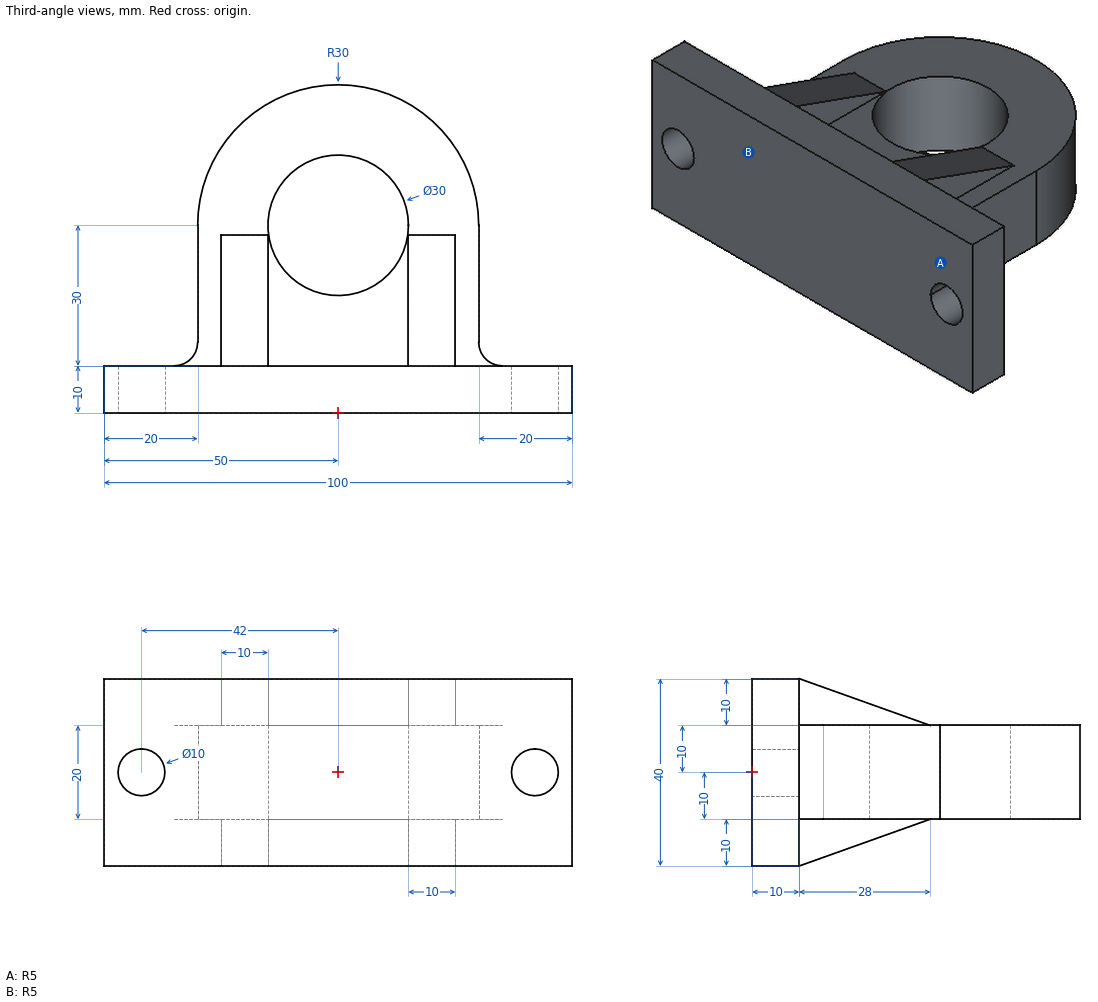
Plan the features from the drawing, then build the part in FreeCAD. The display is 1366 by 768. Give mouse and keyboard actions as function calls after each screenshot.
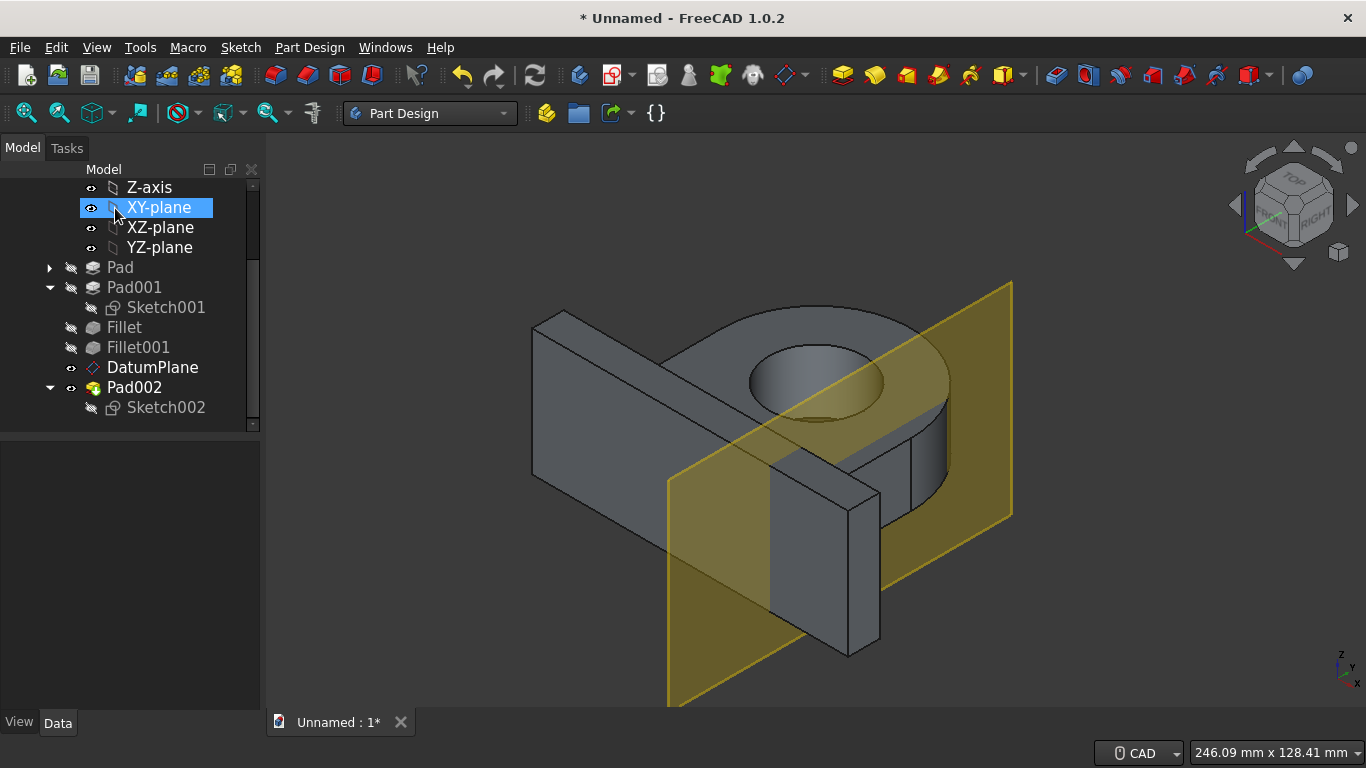
click(116, 368)
key(space)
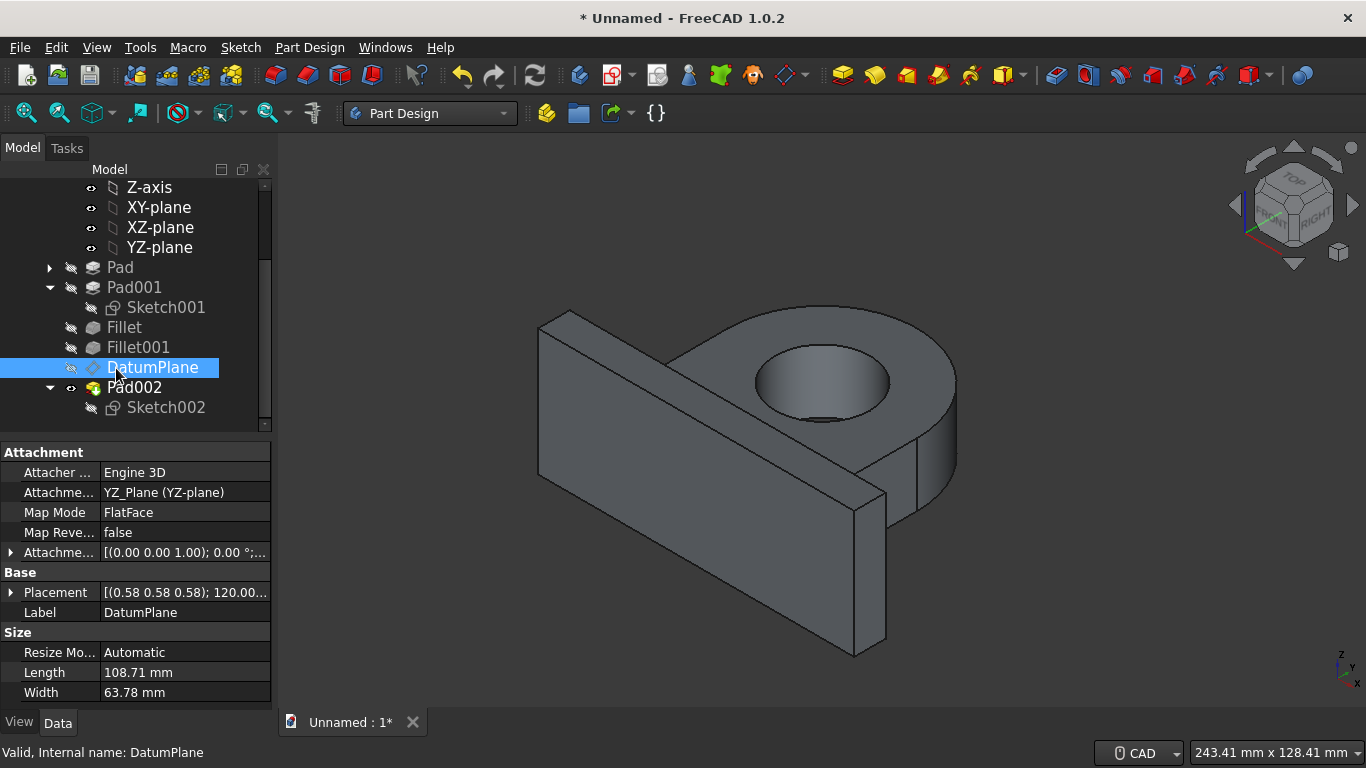
click(116, 388)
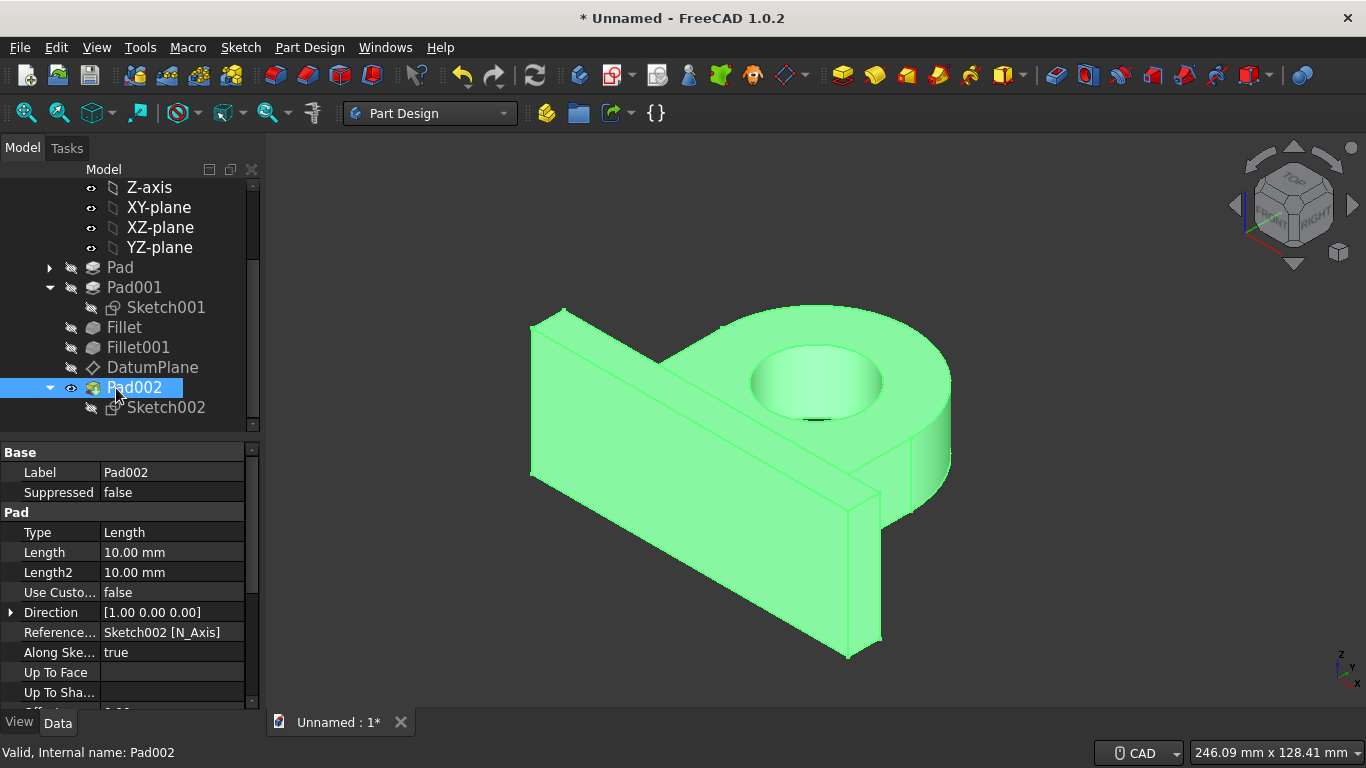
click(136, 76)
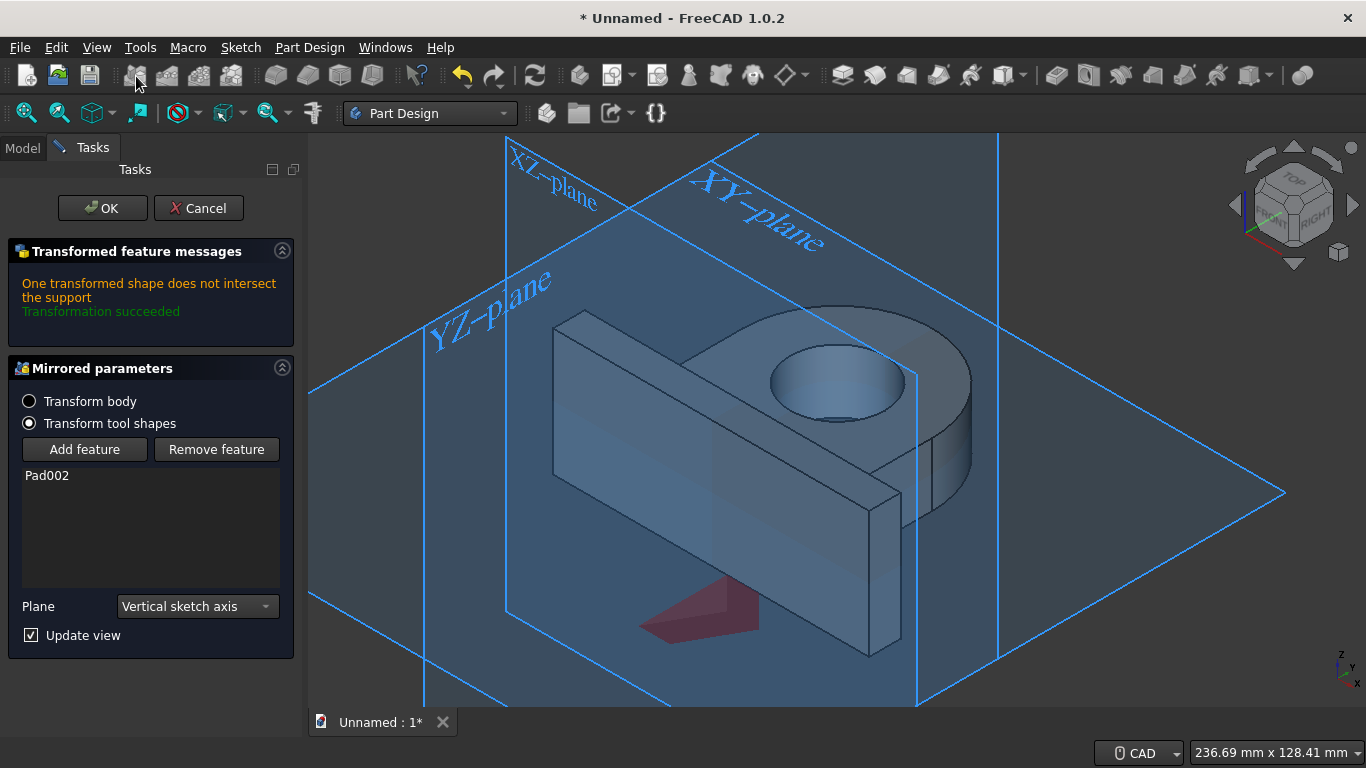
click(198, 606)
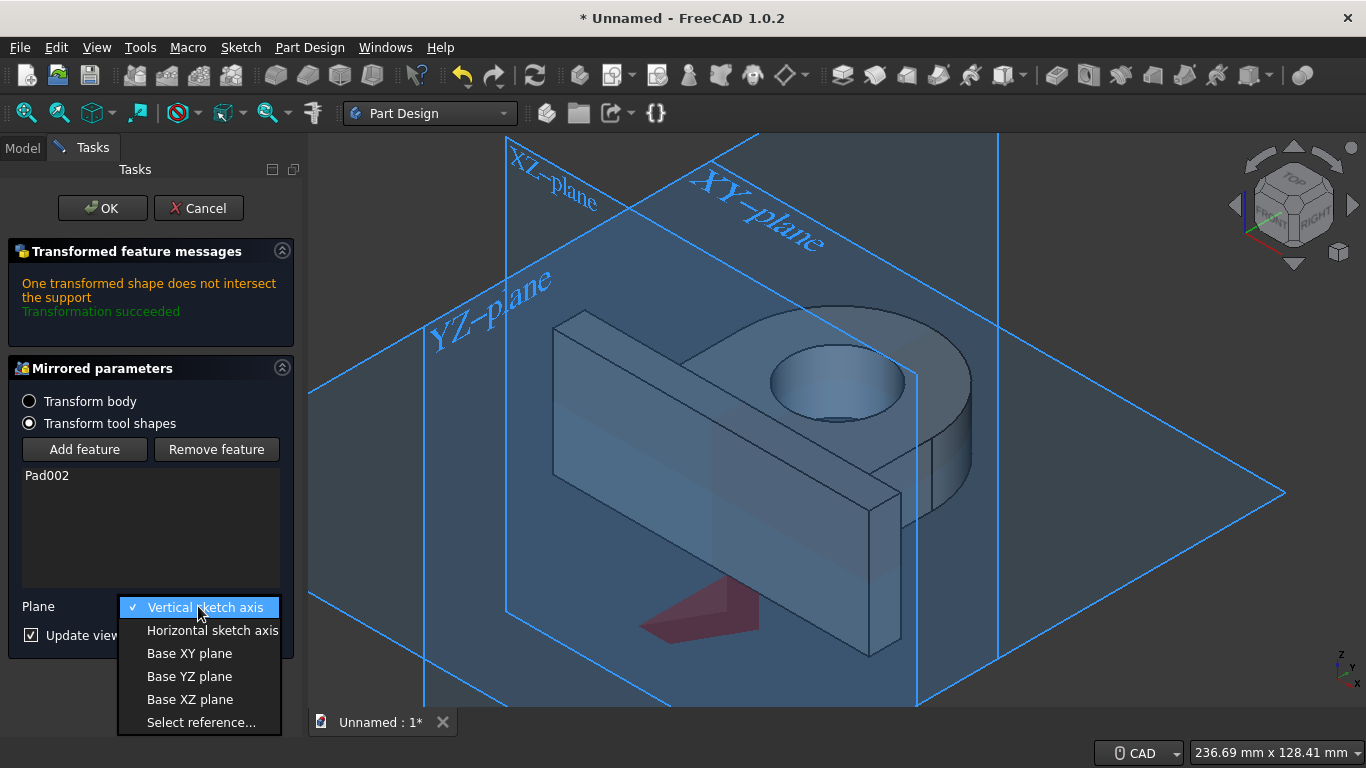
click(198, 676)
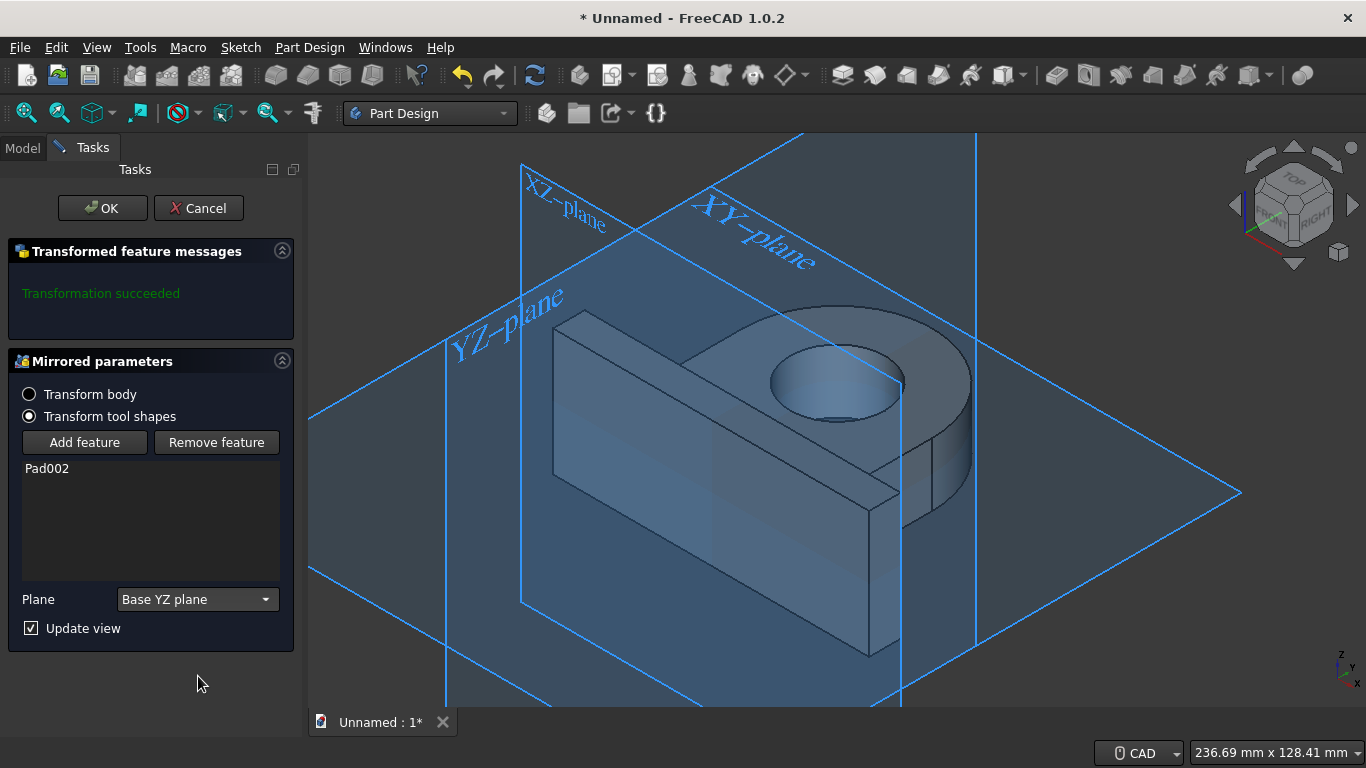
click(103, 208)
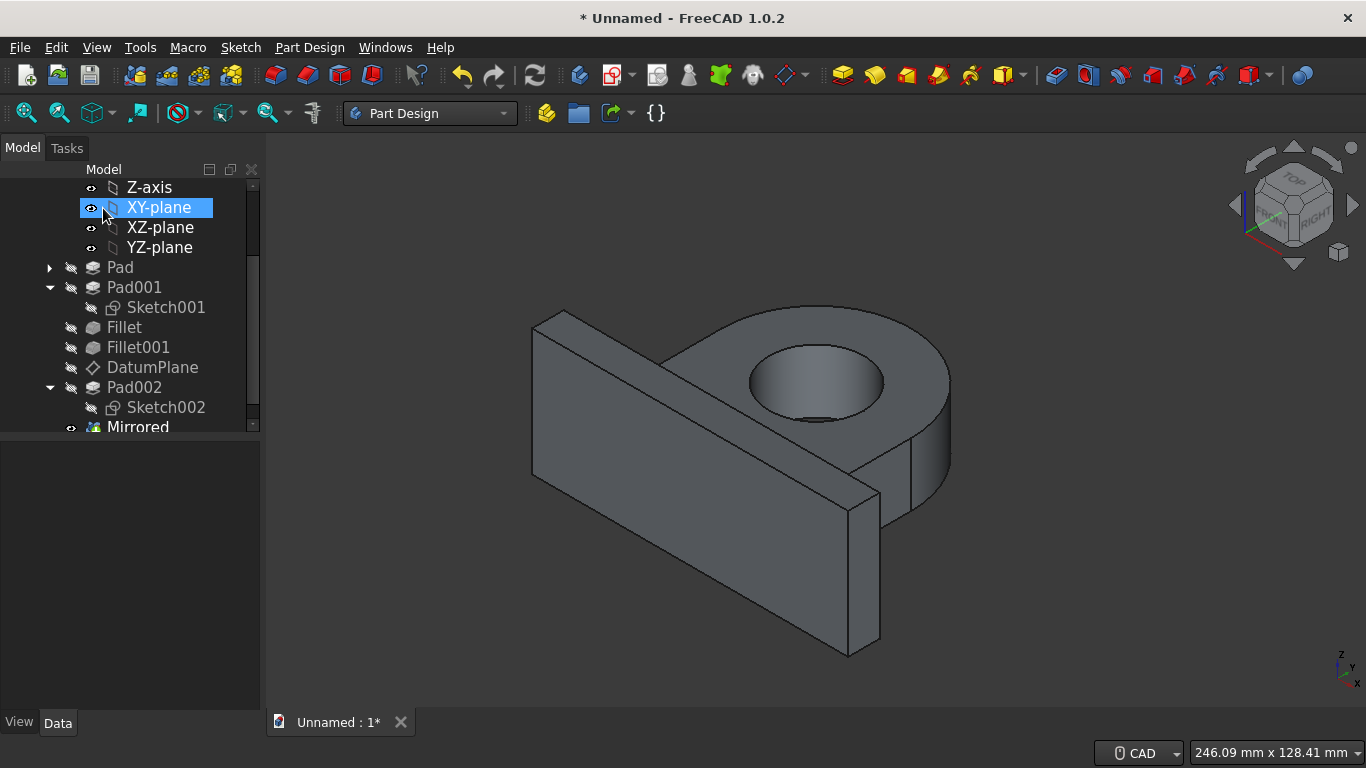
click(116, 388)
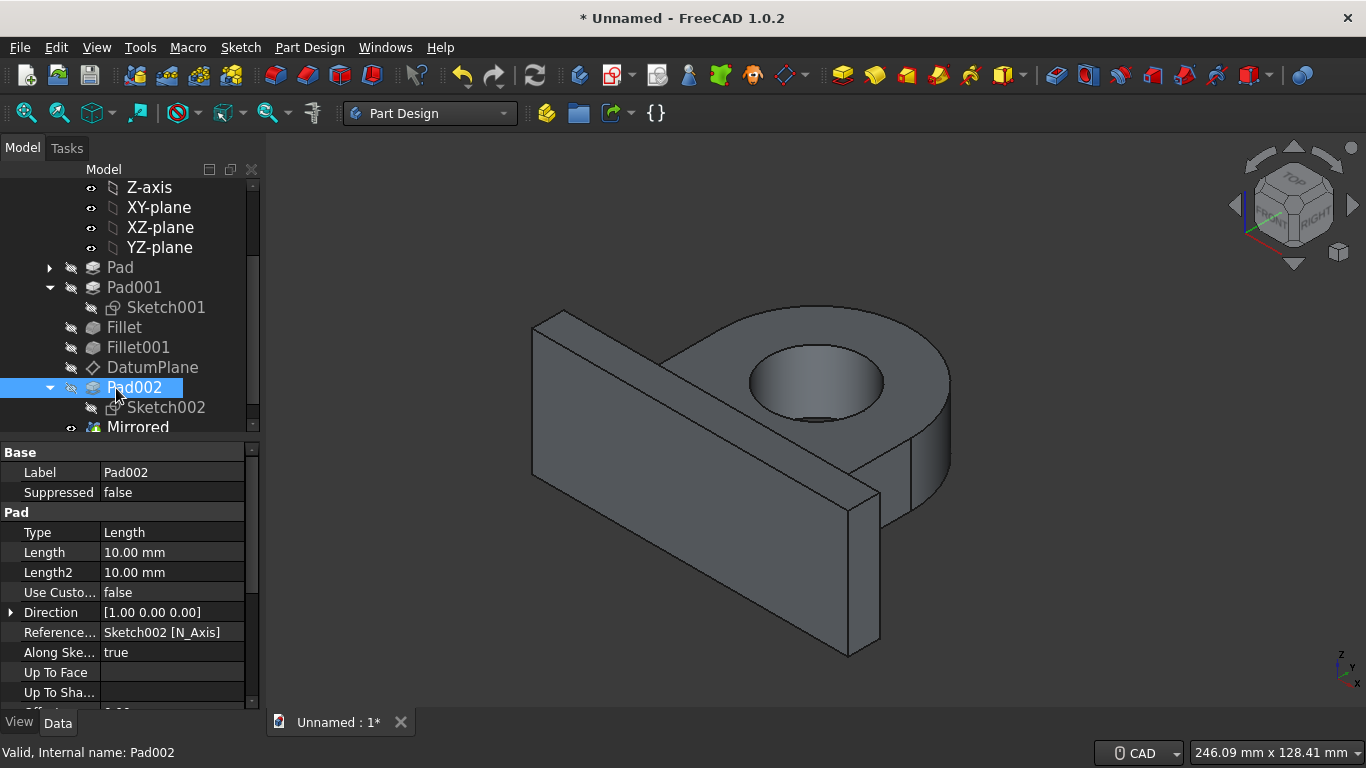
click(136, 76)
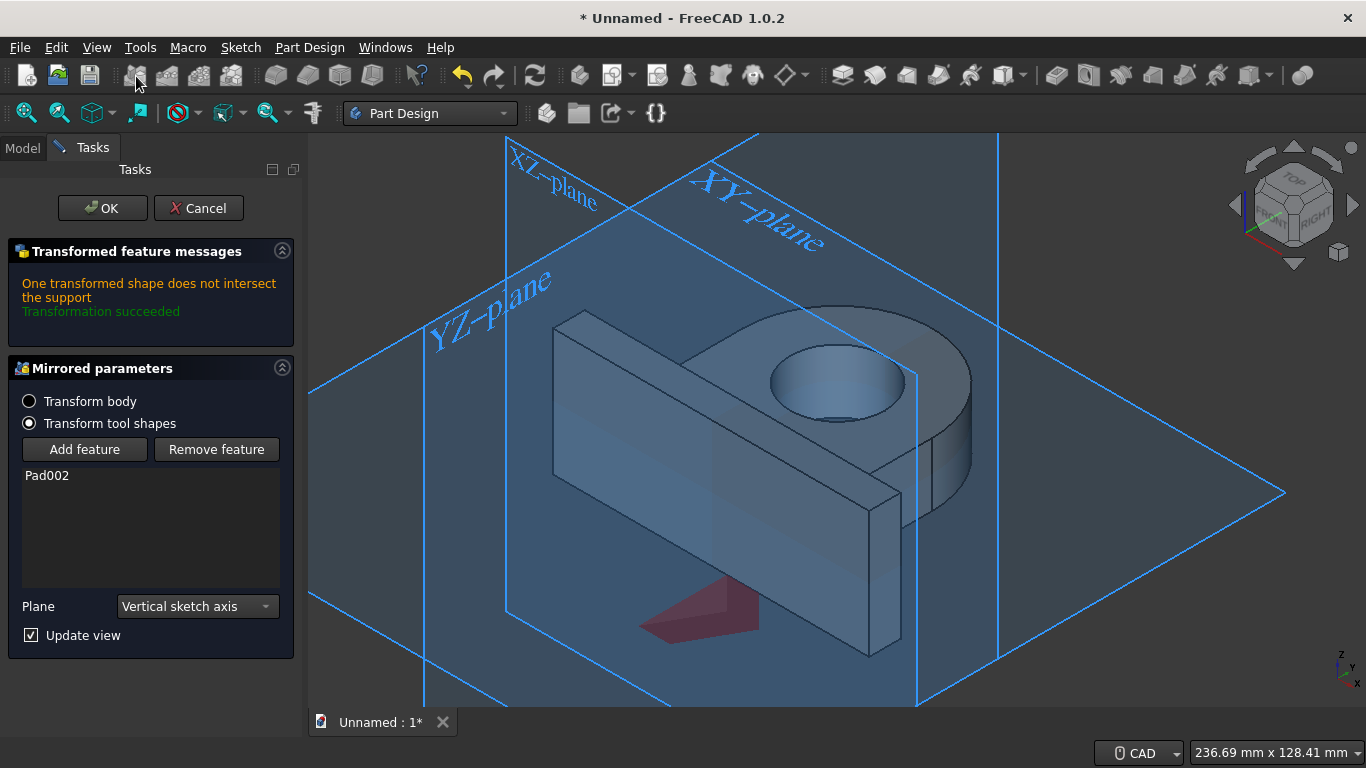
click(198, 606)